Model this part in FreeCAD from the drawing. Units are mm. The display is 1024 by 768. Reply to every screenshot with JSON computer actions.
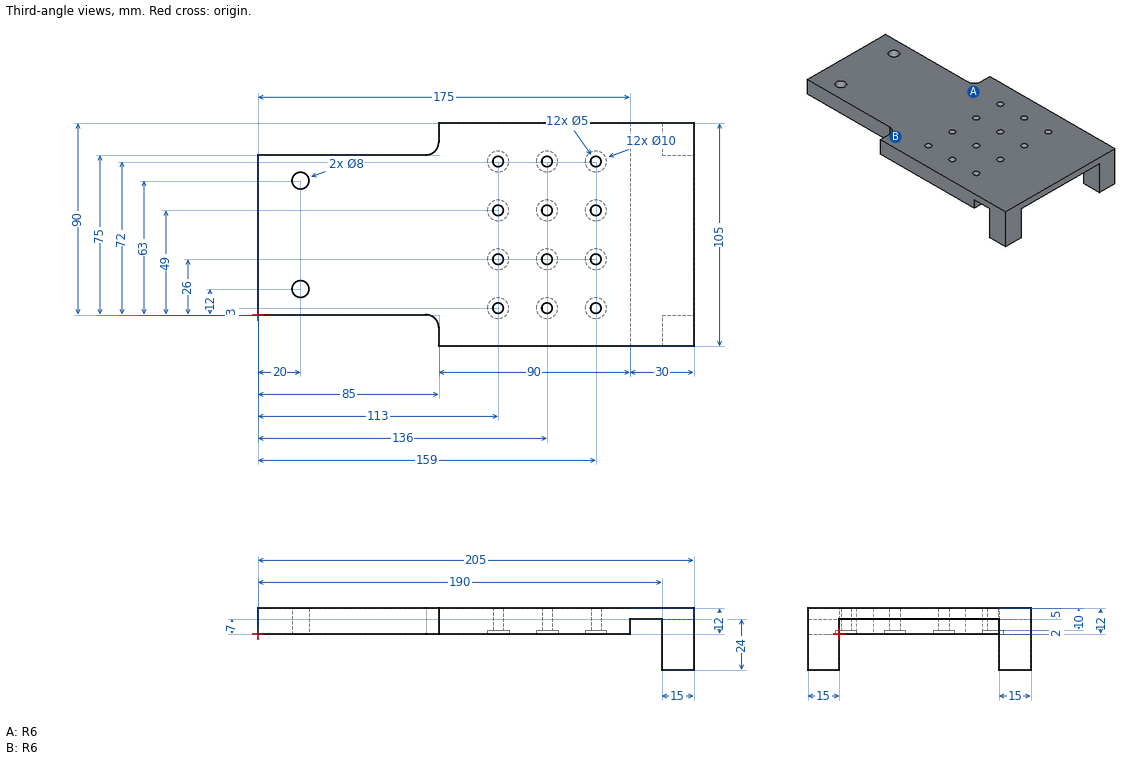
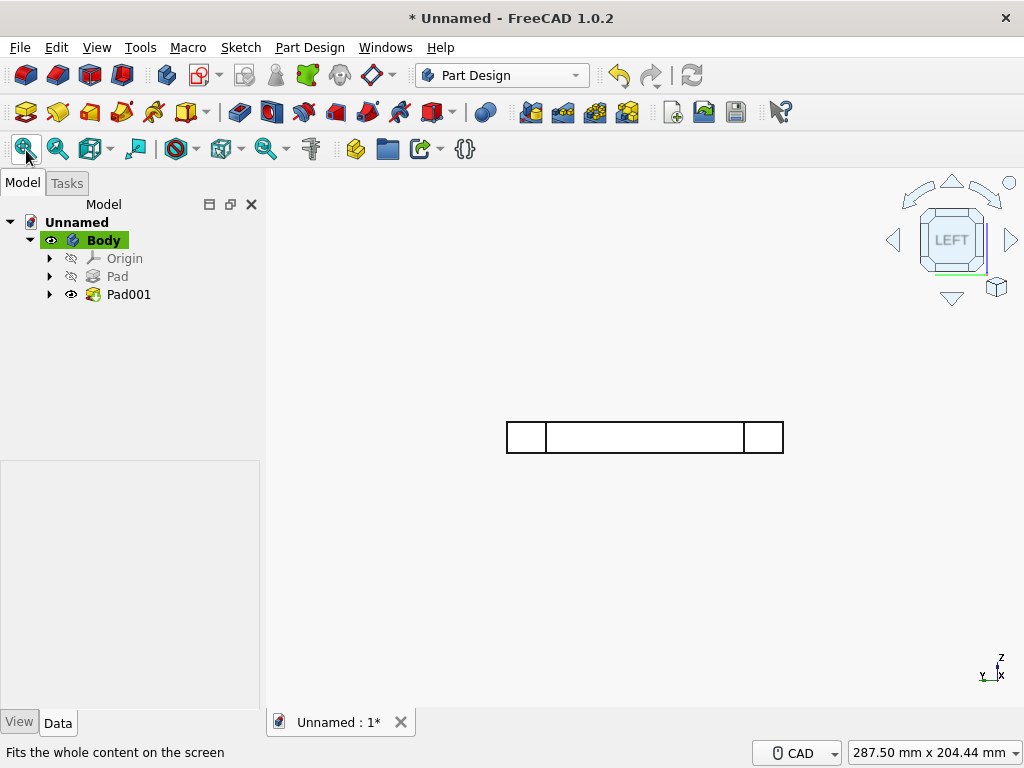
{"action": "key", "text": "v 3"}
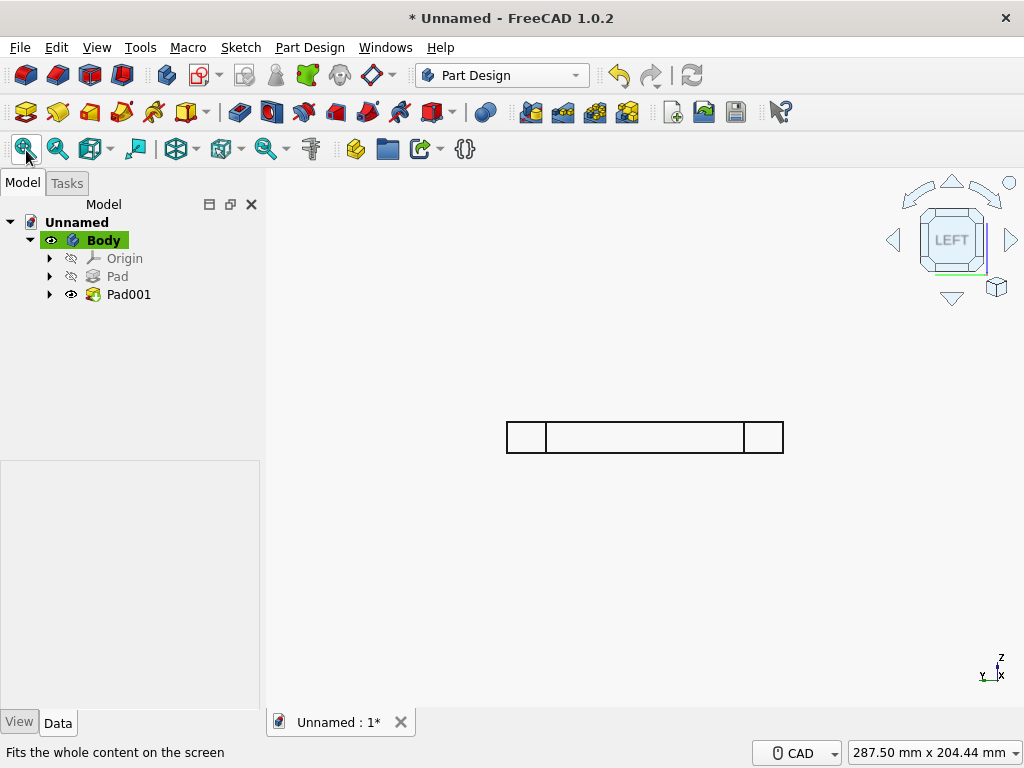
{"action": "key", "text": "0"}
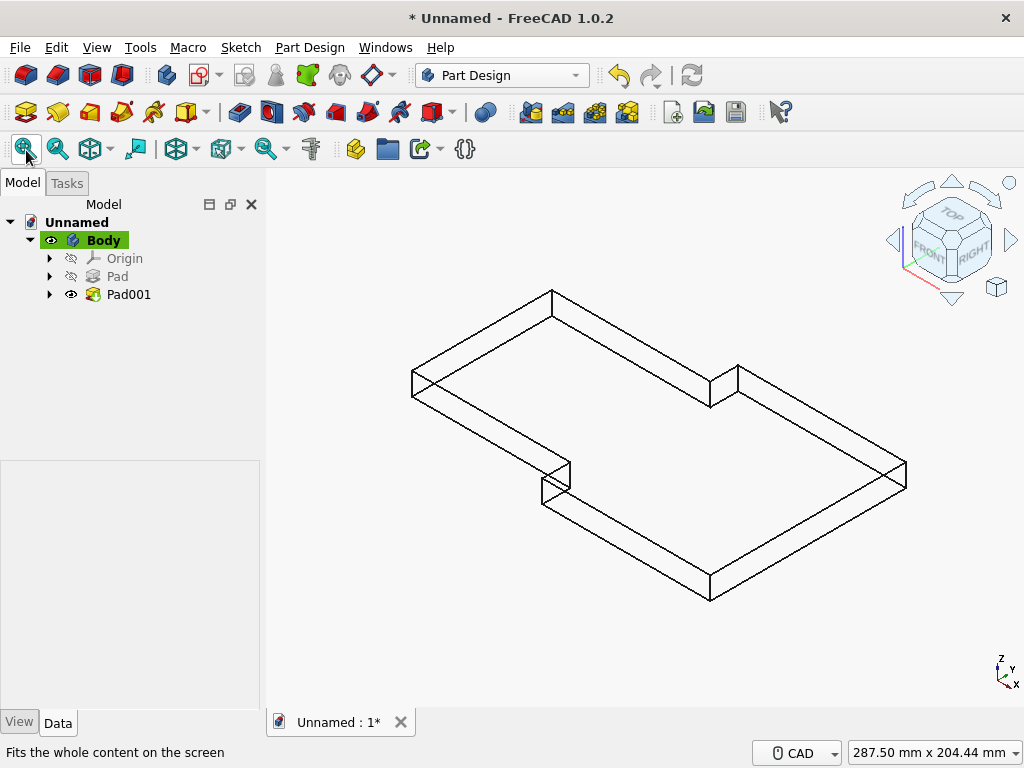
{"action": "left_click", "coordinate": [710, 393]}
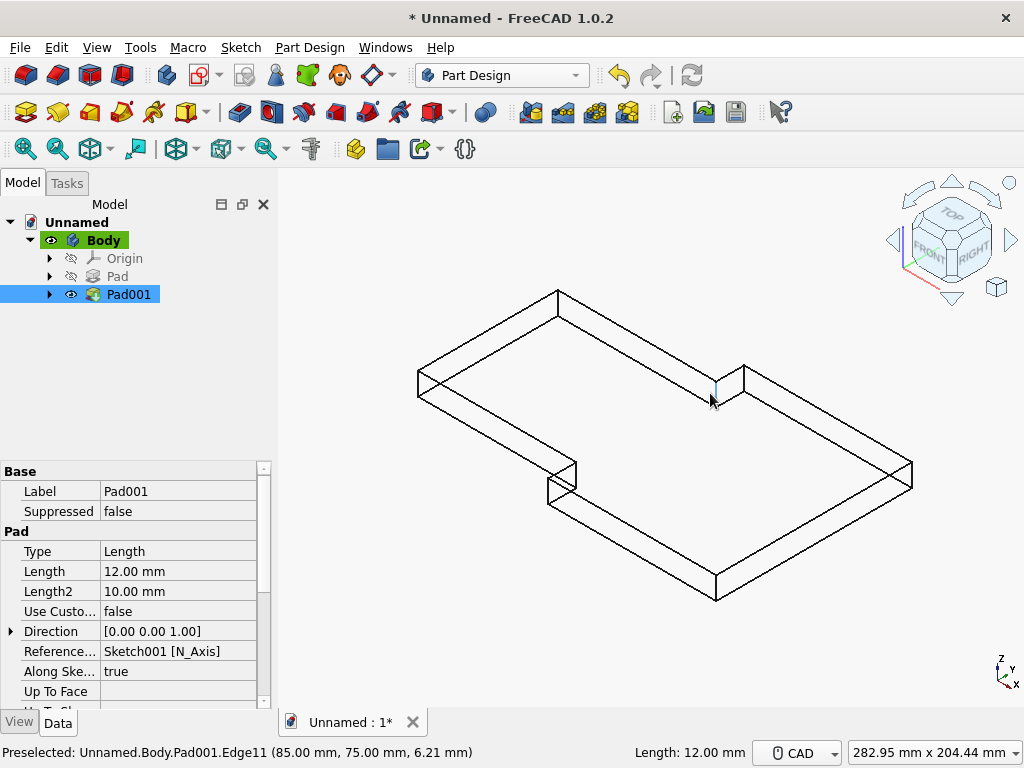
{"action": "key", "text": "v 1"}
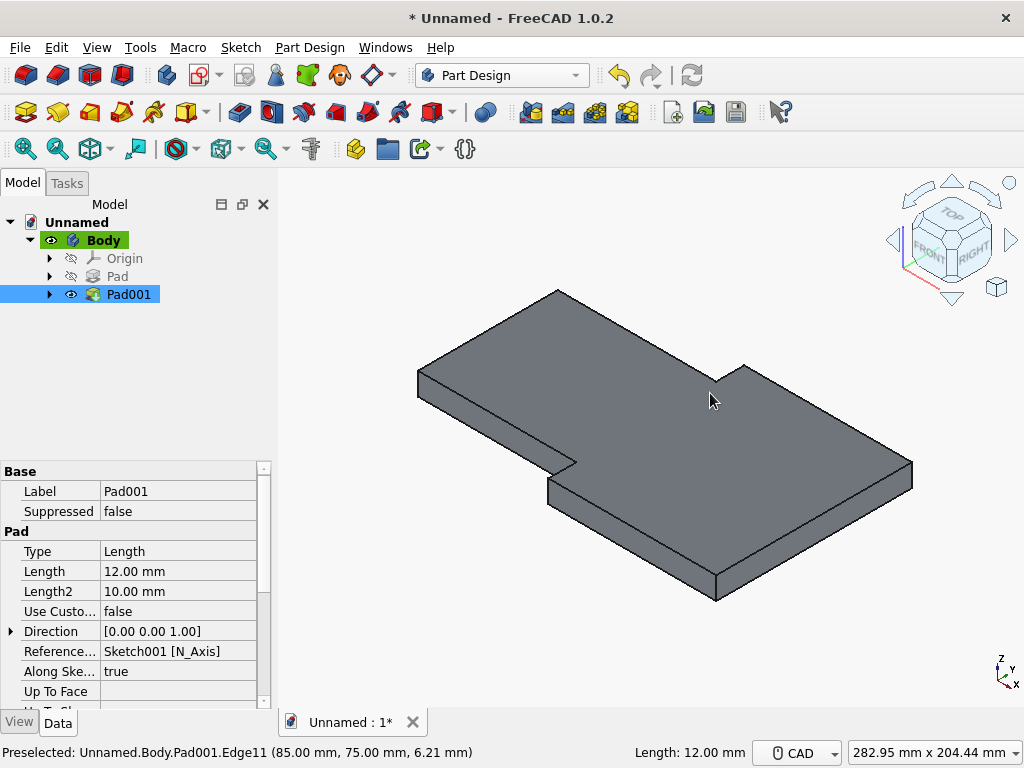
{"action": "left_click", "coordinate": [26, 76]}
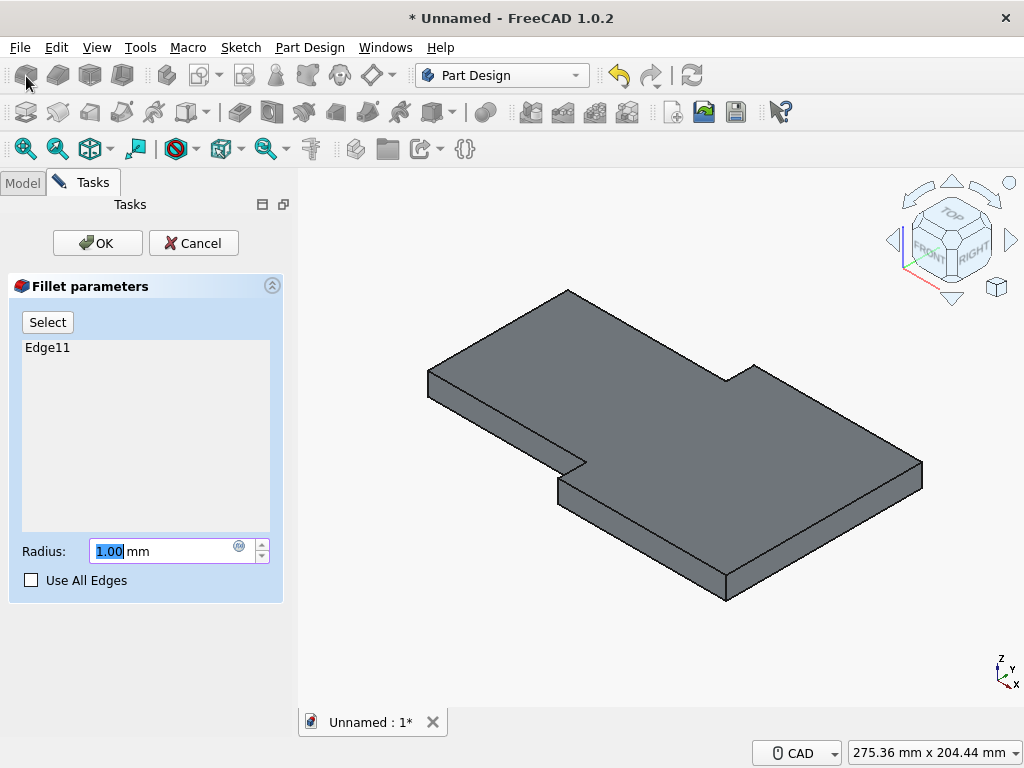
{"action": "type", "text": "6"}
{"action": "key", "text": "Tab"}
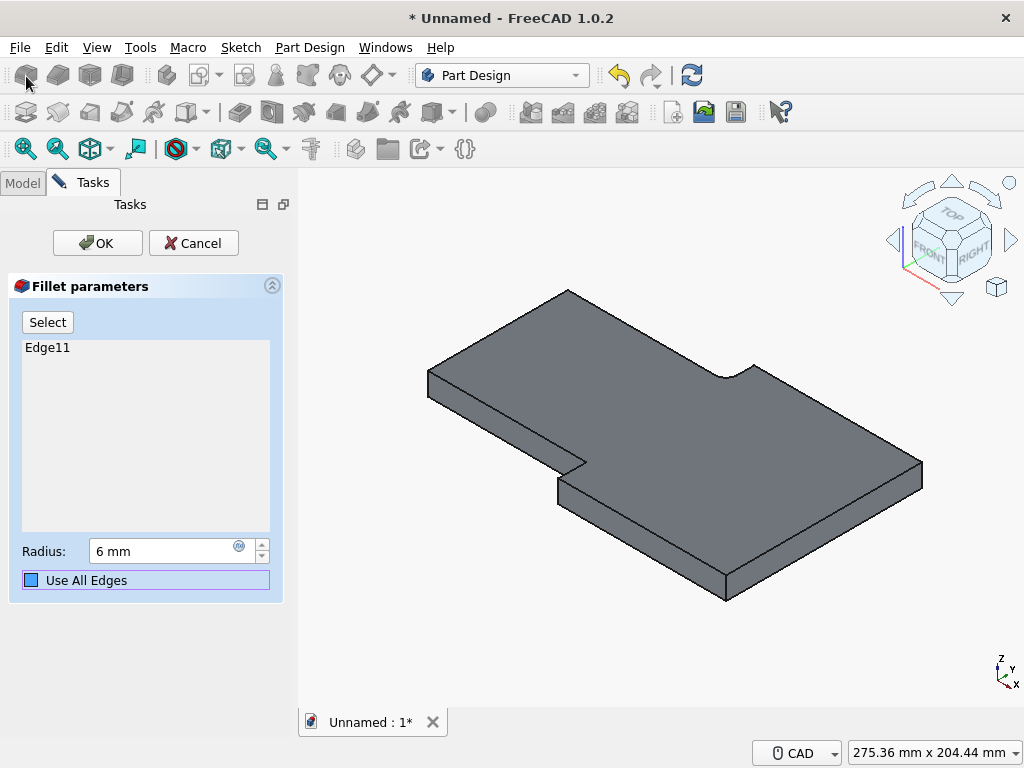
{"action": "left_click", "coordinate": [98, 243]}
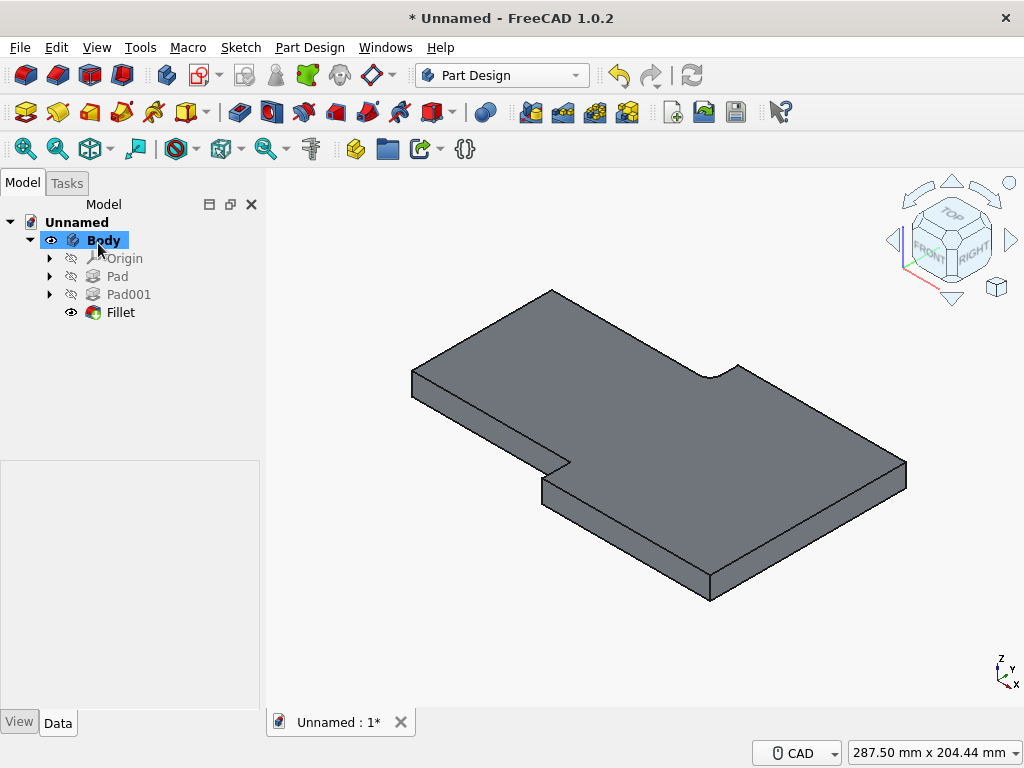
{"action": "key", "text": "2"}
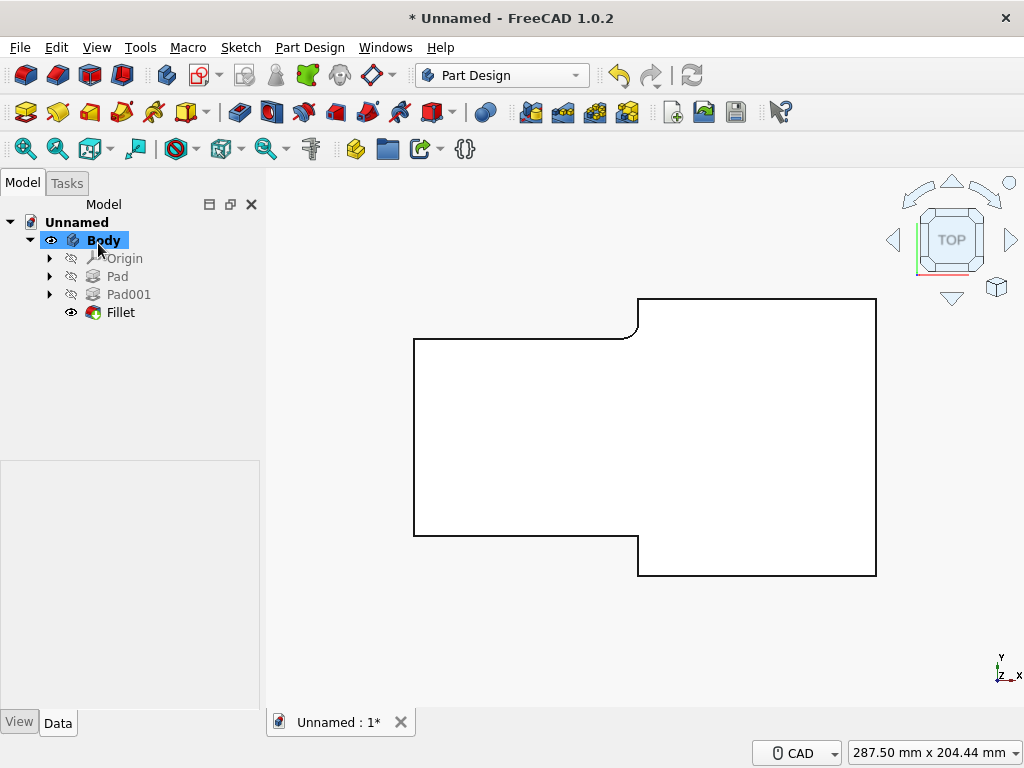
{"action": "key", "text": "0"}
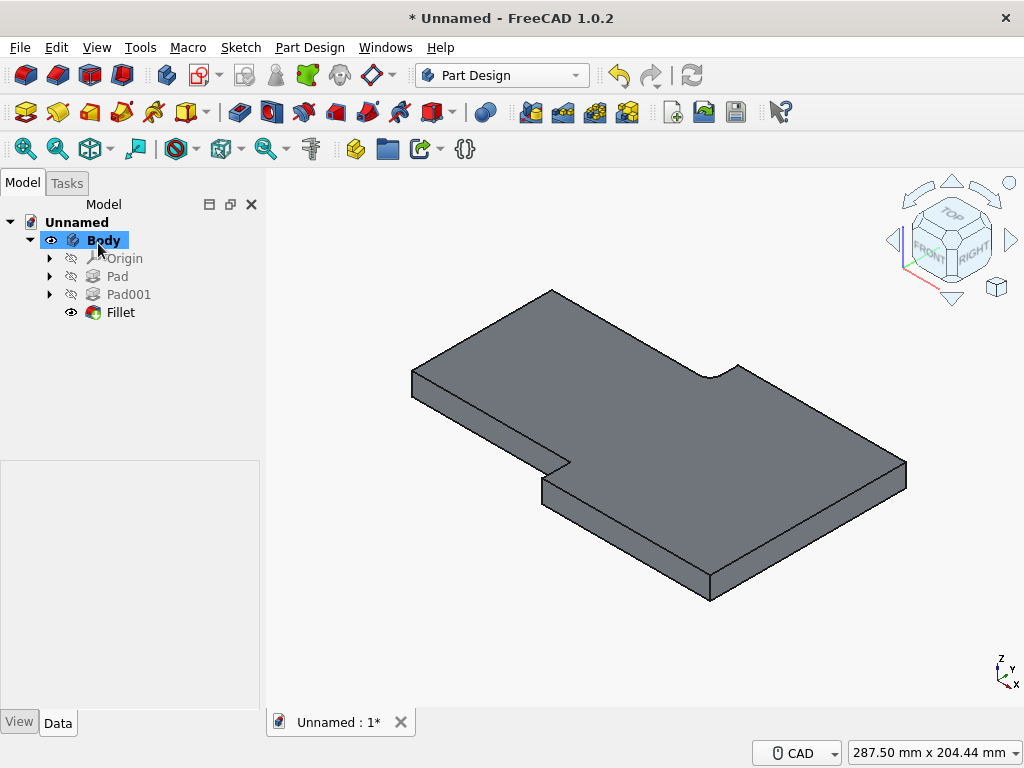
{"action": "key", "text": "1"}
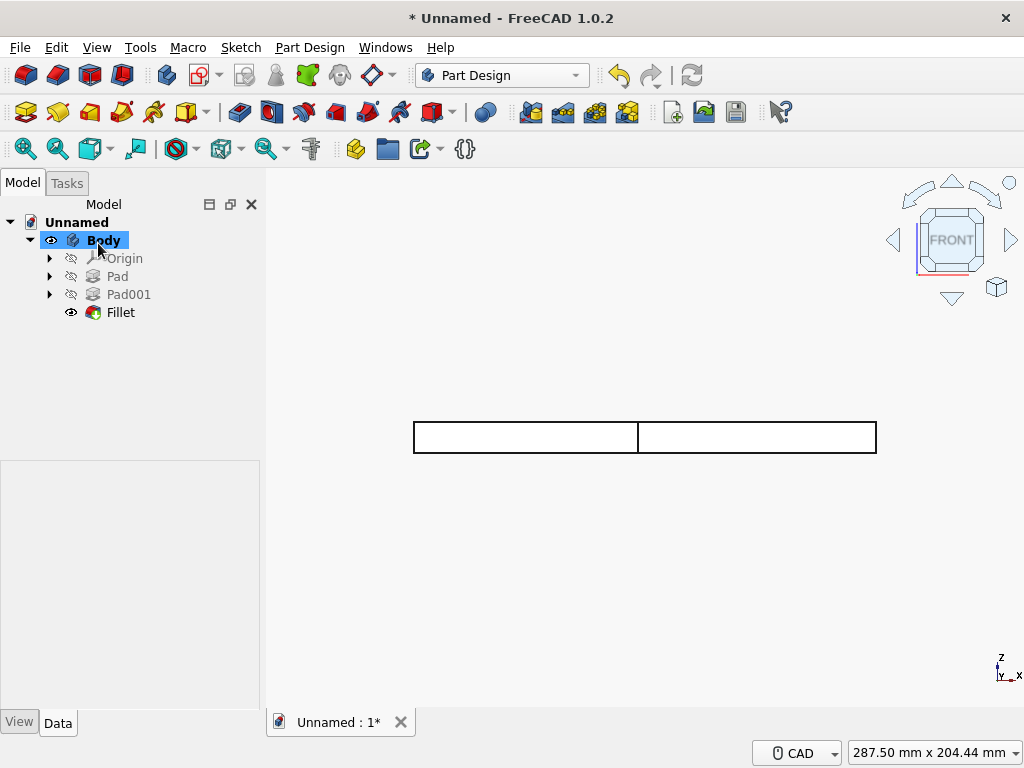
{"action": "key", "text": "3"}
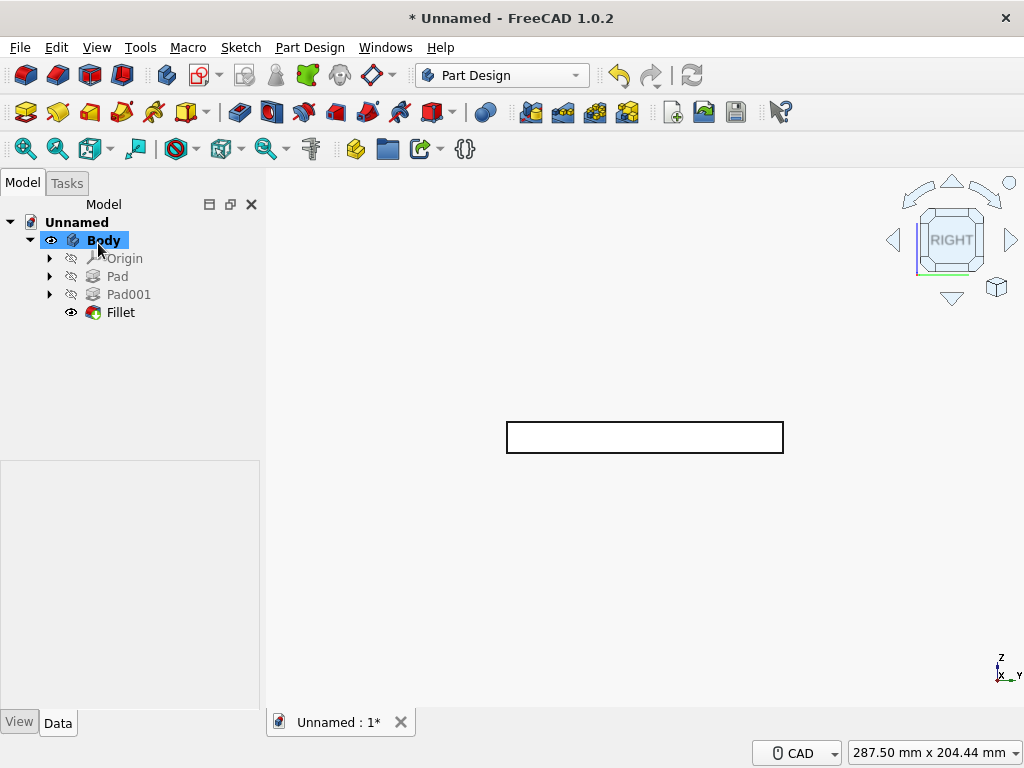
{"action": "left_click", "coordinate": [26, 150]}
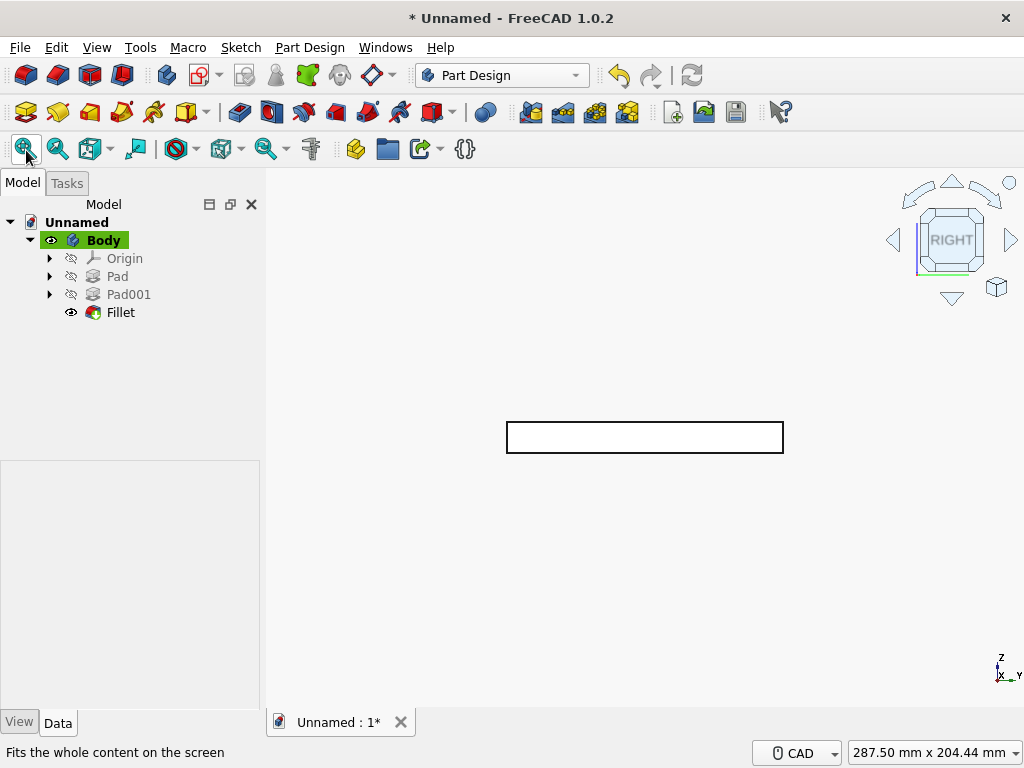
{"action": "key", "text": "5"}